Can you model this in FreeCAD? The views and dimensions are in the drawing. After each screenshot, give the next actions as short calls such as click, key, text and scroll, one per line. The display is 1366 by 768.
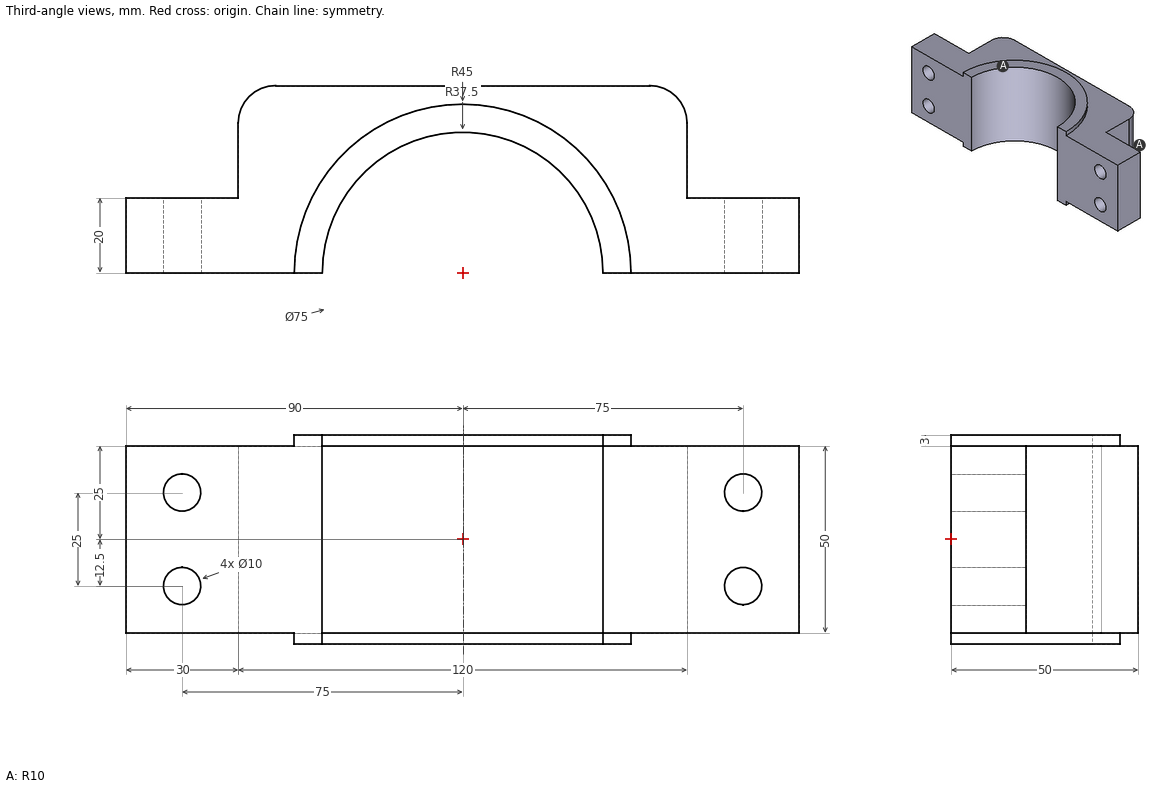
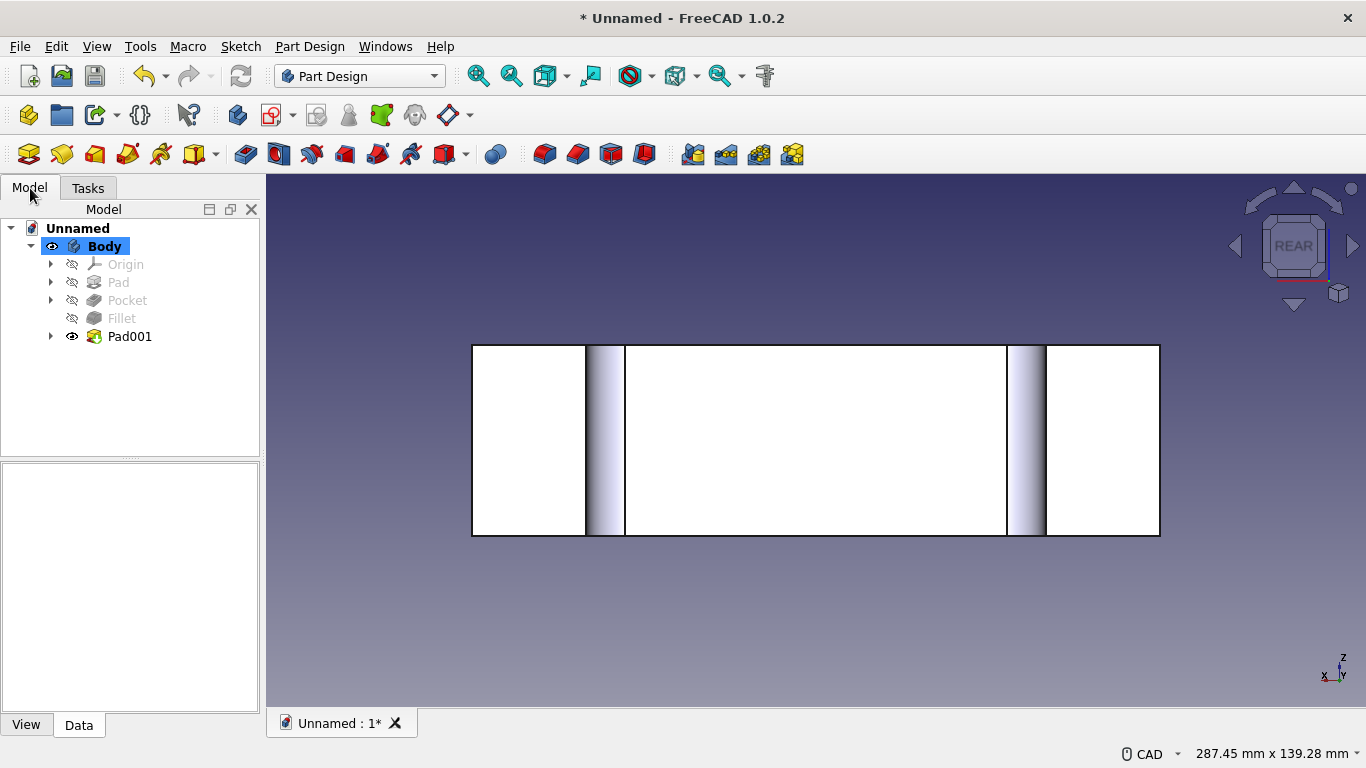
click(51, 264)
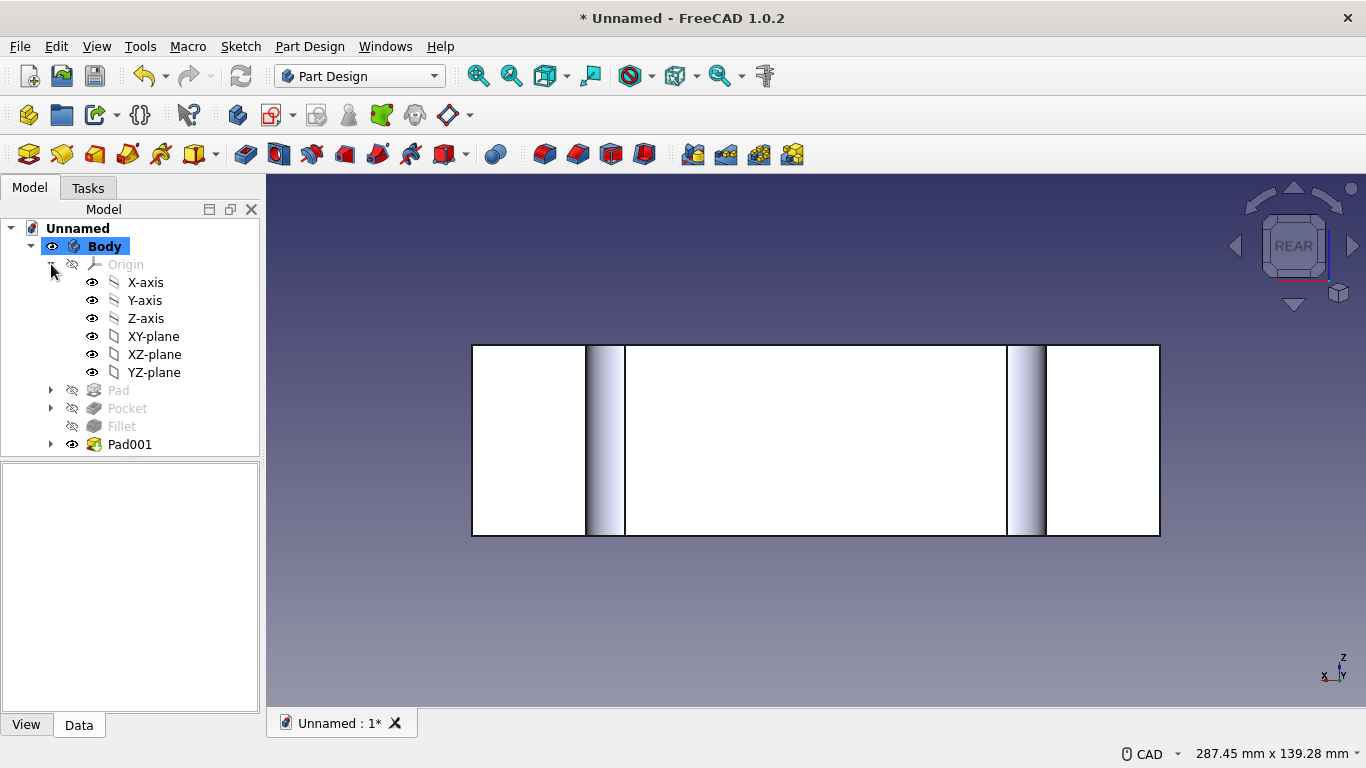
click(137, 336)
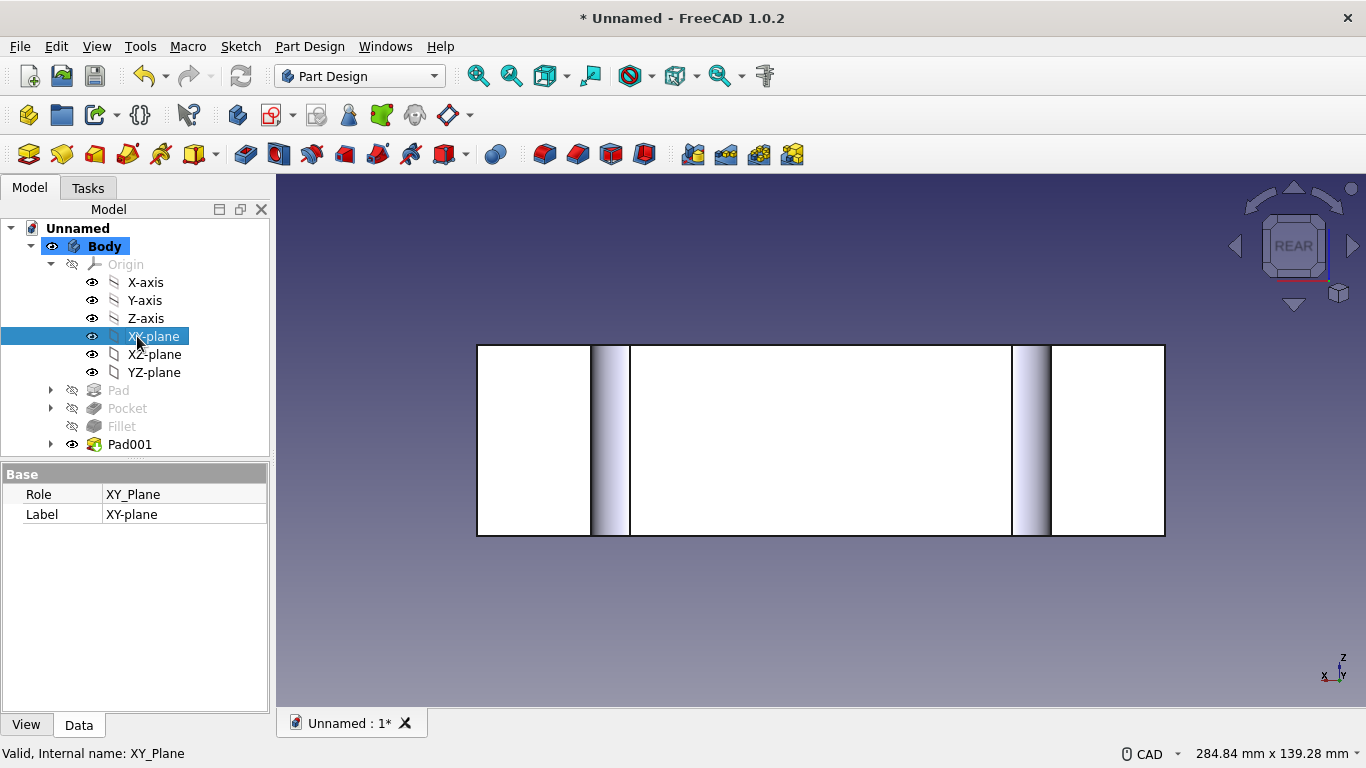
click(448, 116)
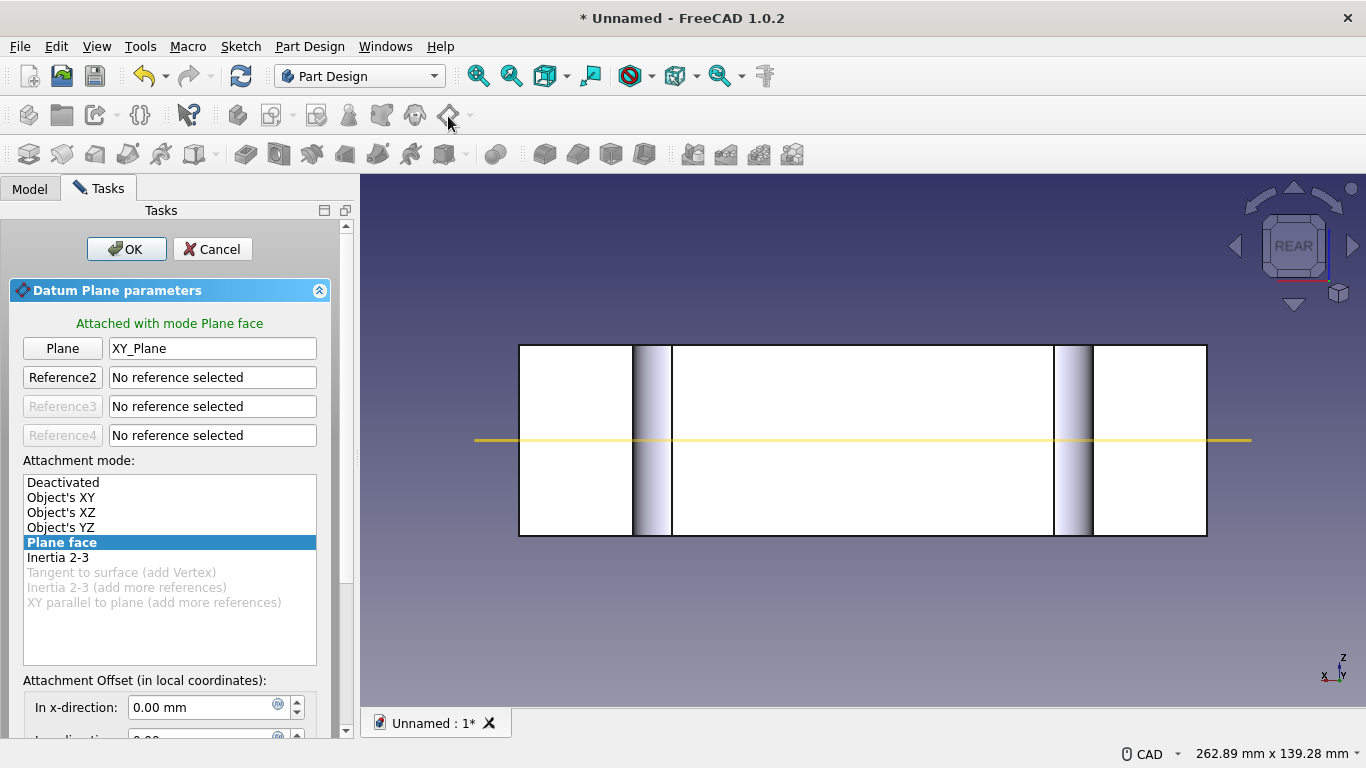
scroll(346, 479, down, 2)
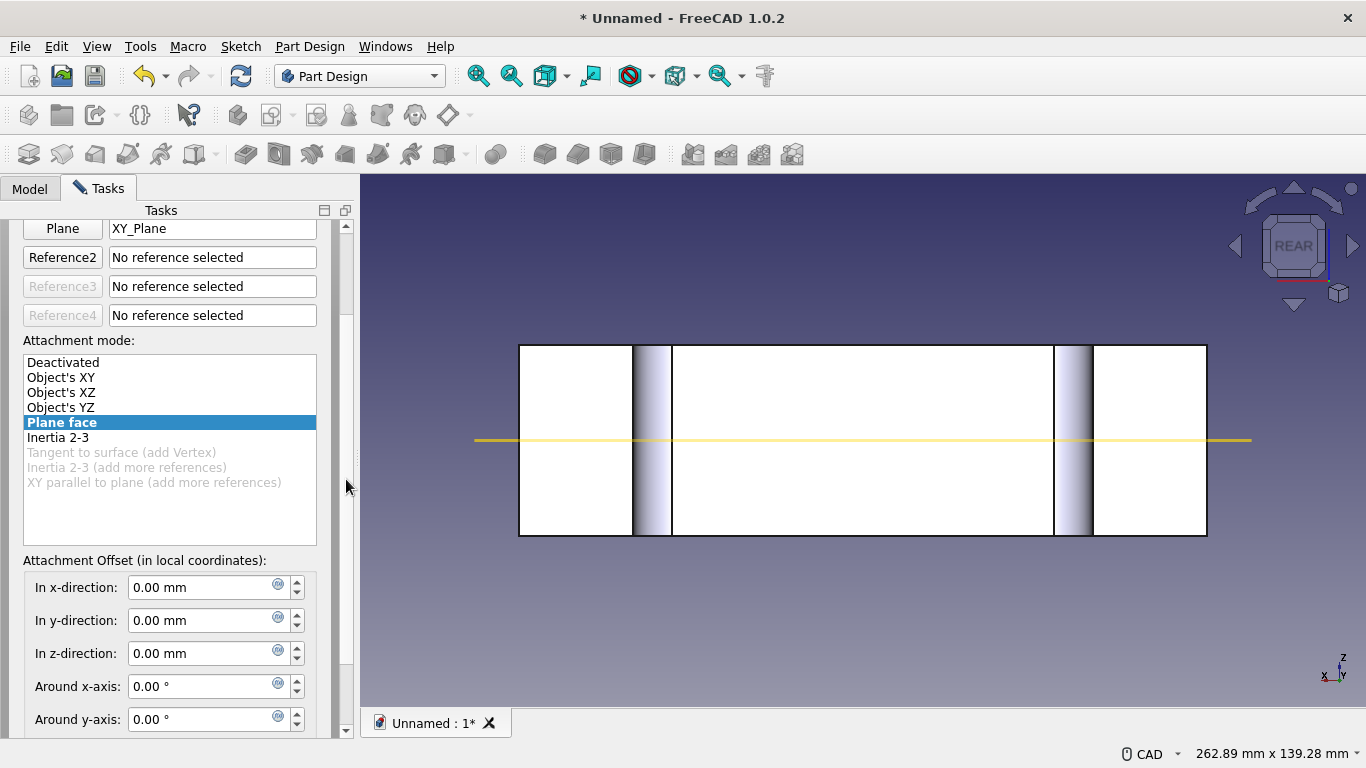
triple_click(210, 654)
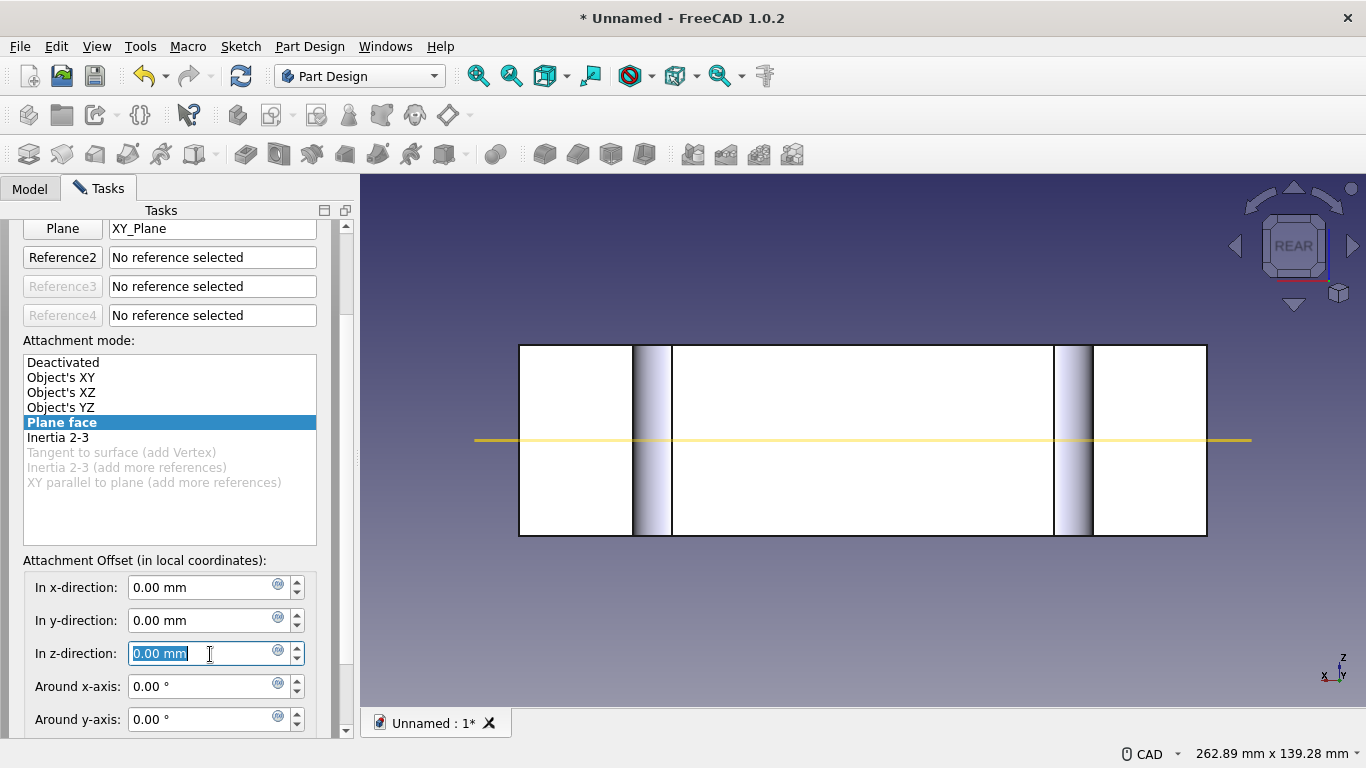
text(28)
key(Tab)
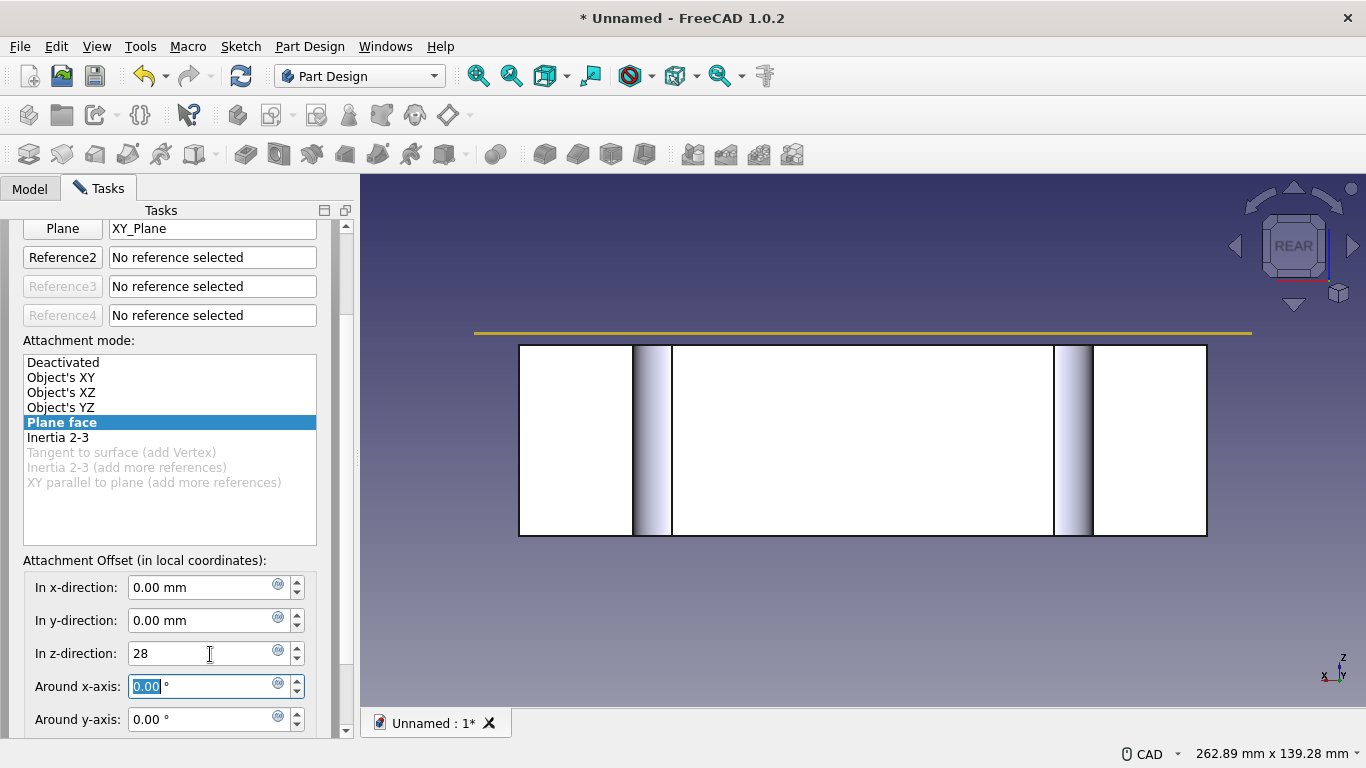
scroll(346, 479, up, 3)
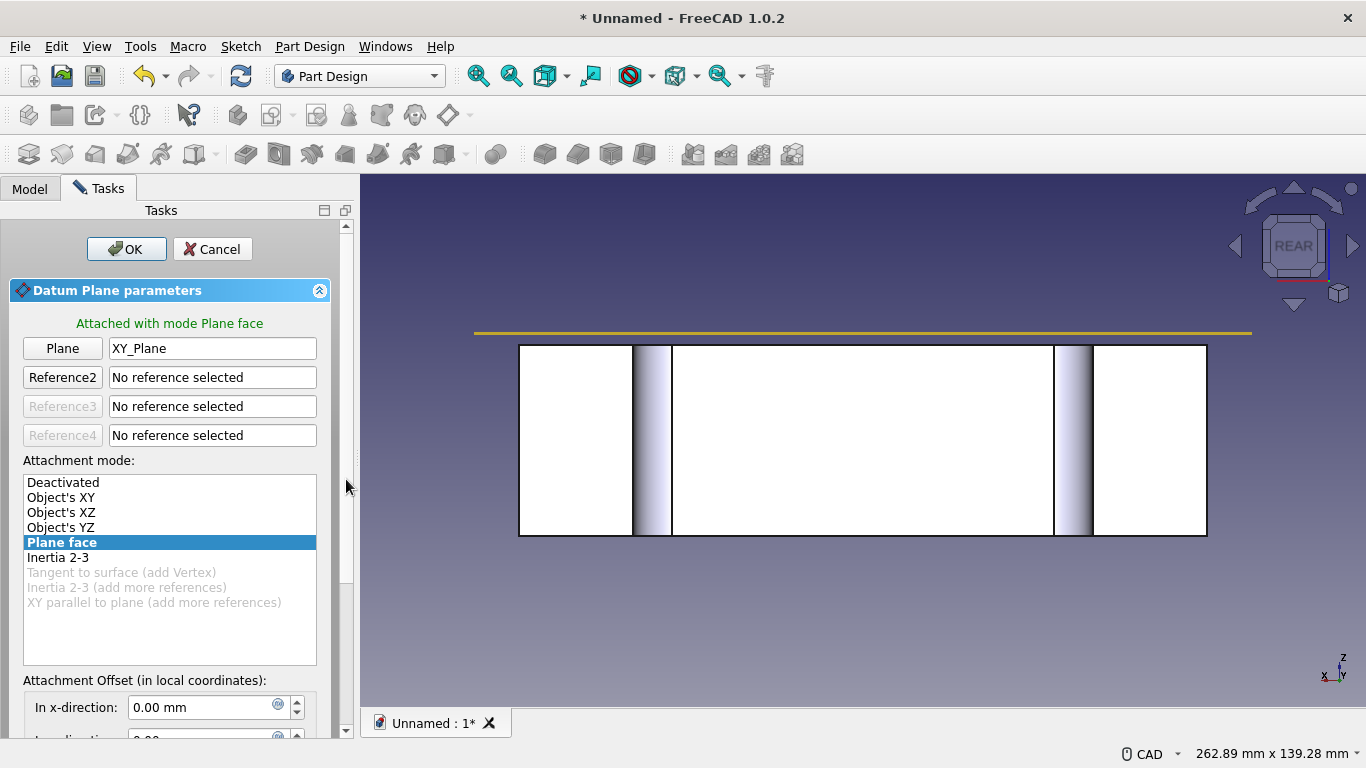
click(127, 249)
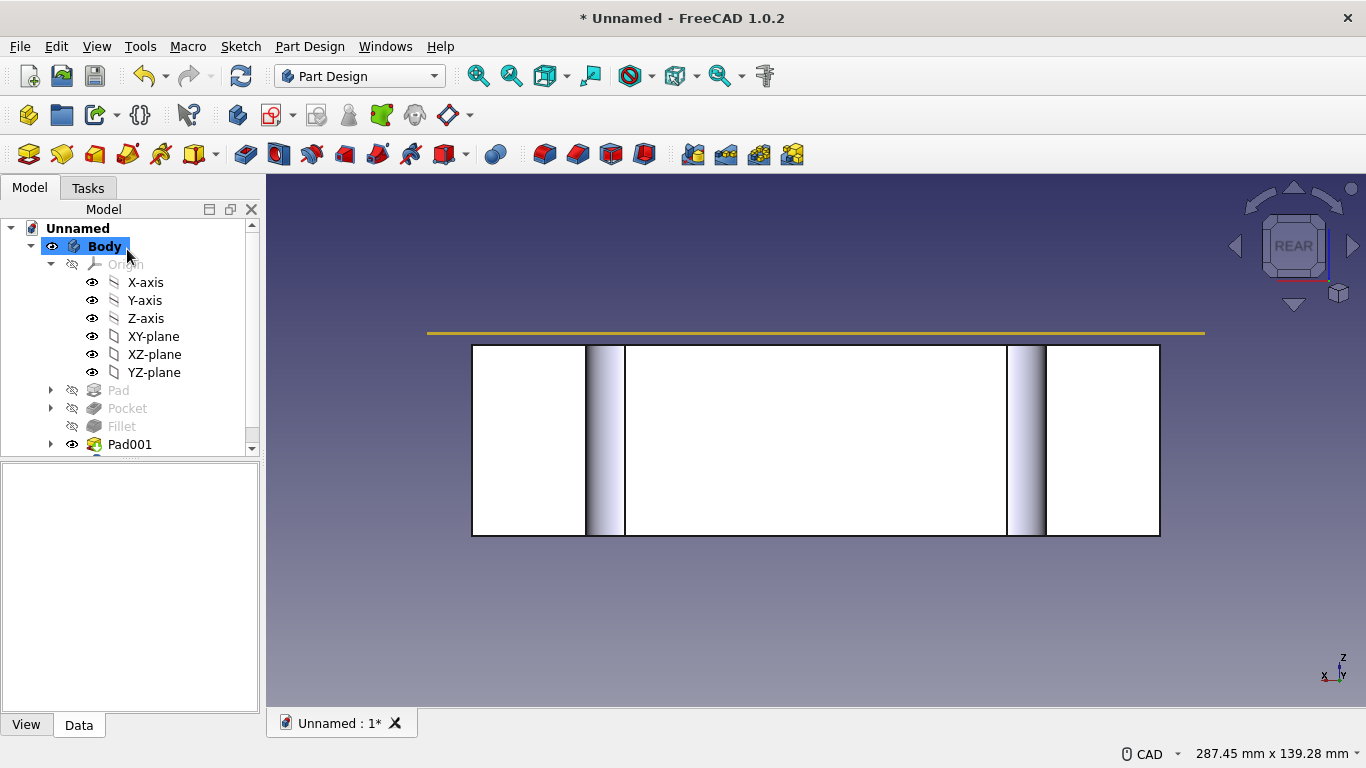
scroll(101, 332, down, 3)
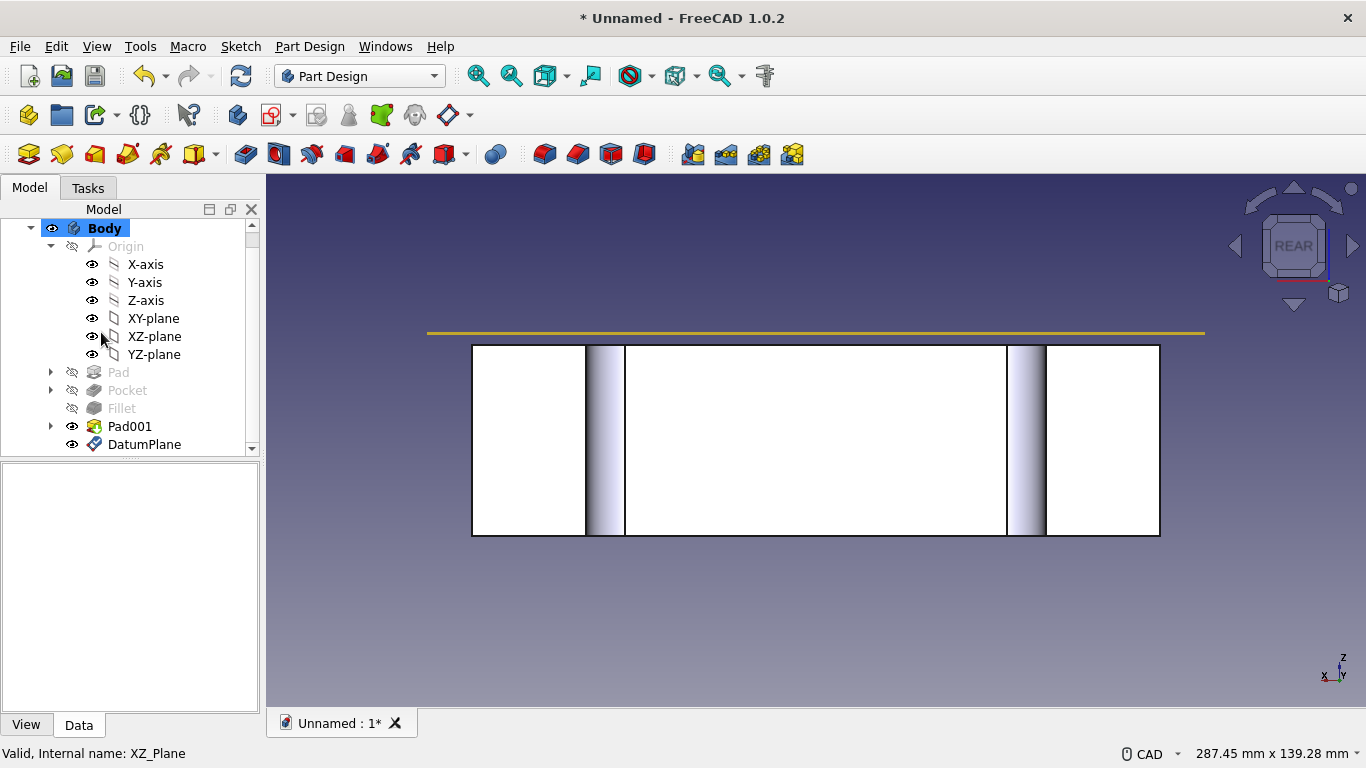
click(117, 444)